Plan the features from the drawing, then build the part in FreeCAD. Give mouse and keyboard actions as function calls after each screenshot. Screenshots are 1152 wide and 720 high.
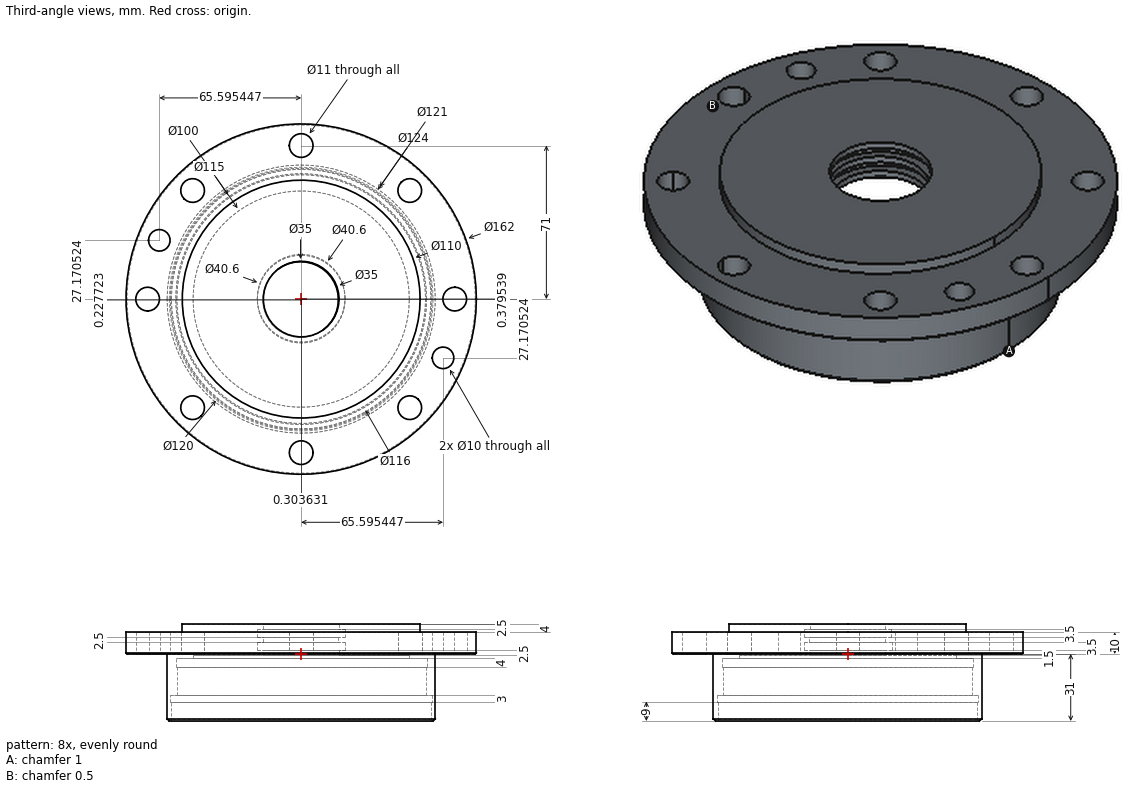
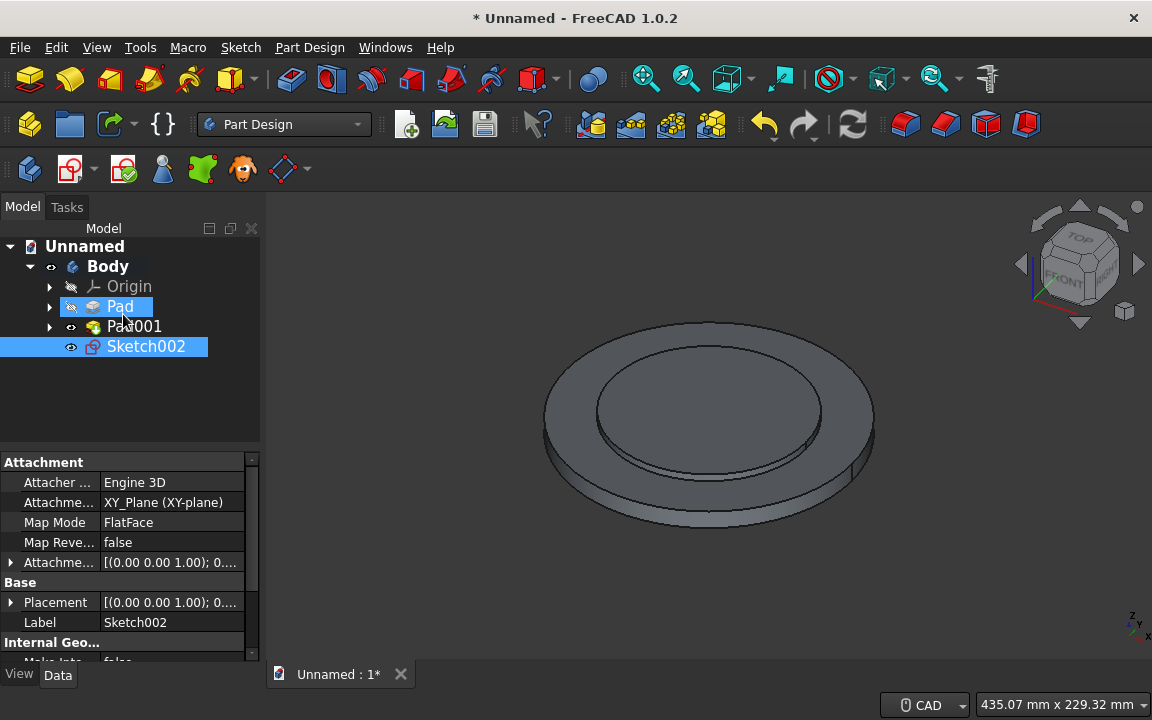
click(30, 80)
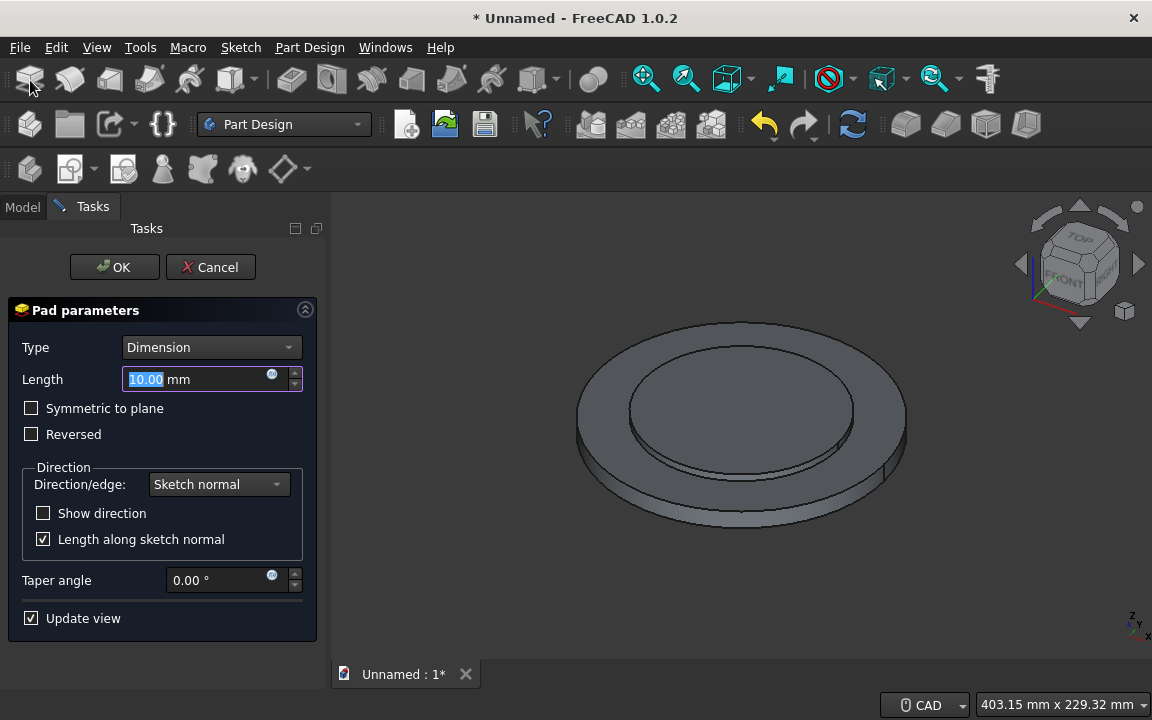
text(31)
key(Tab)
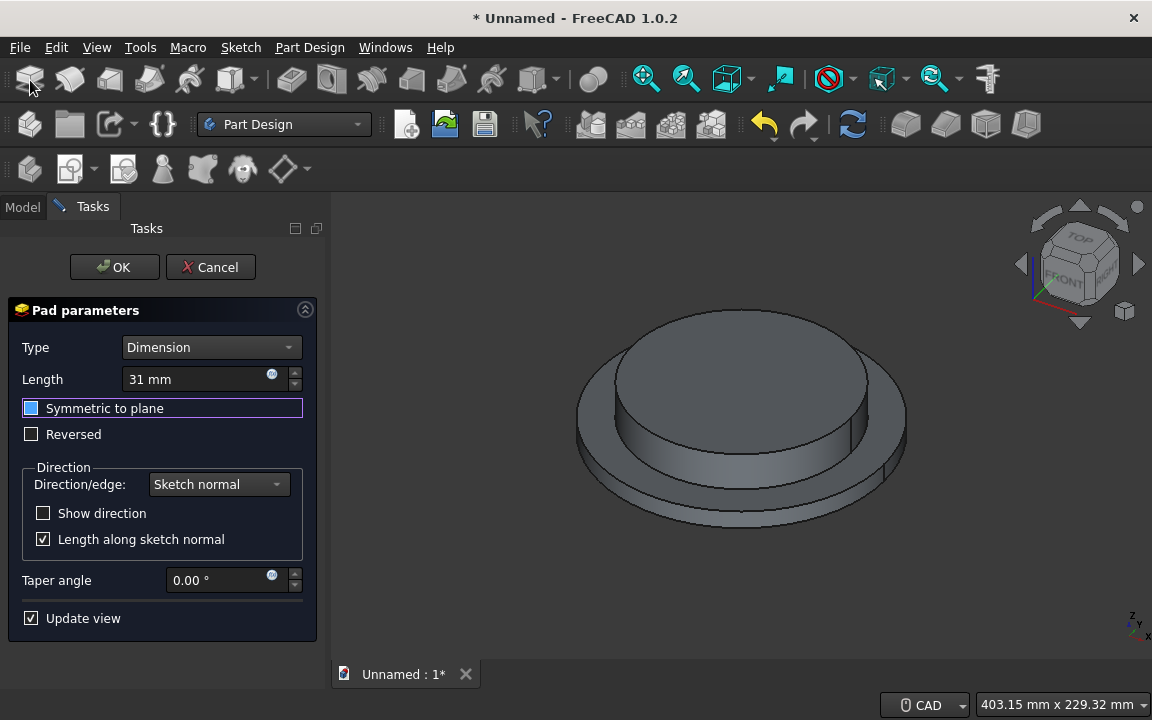
click(30, 434)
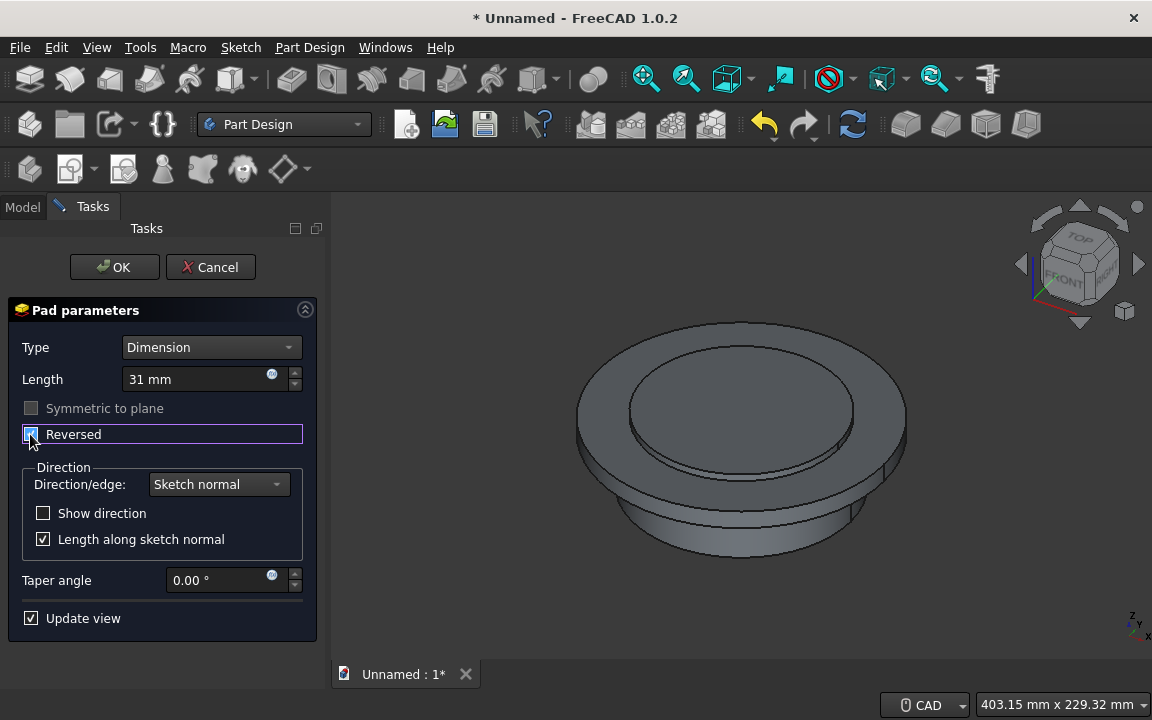
click(115, 267)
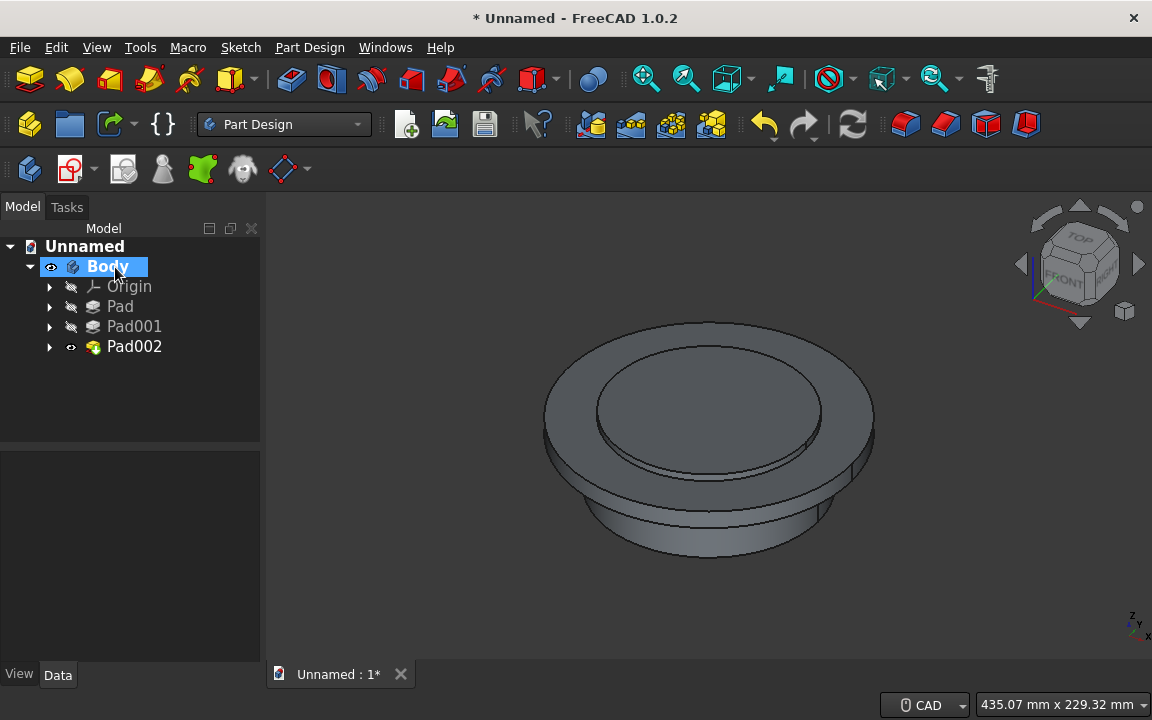
click(709, 409)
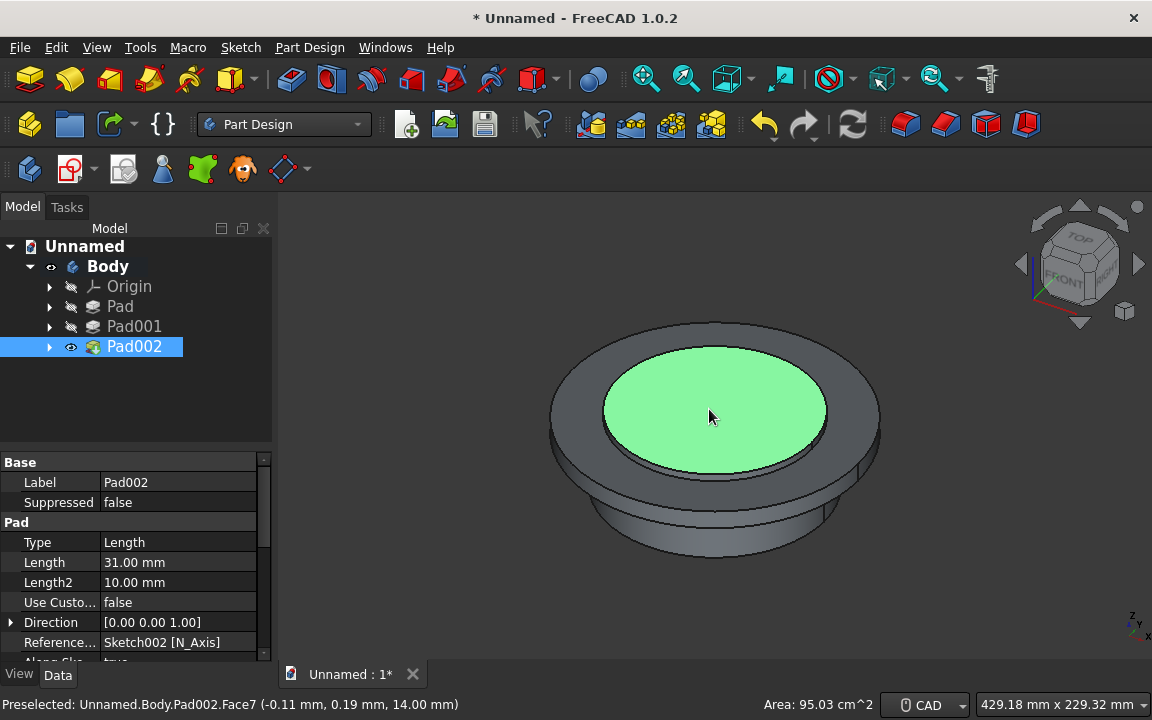
click(70, 170)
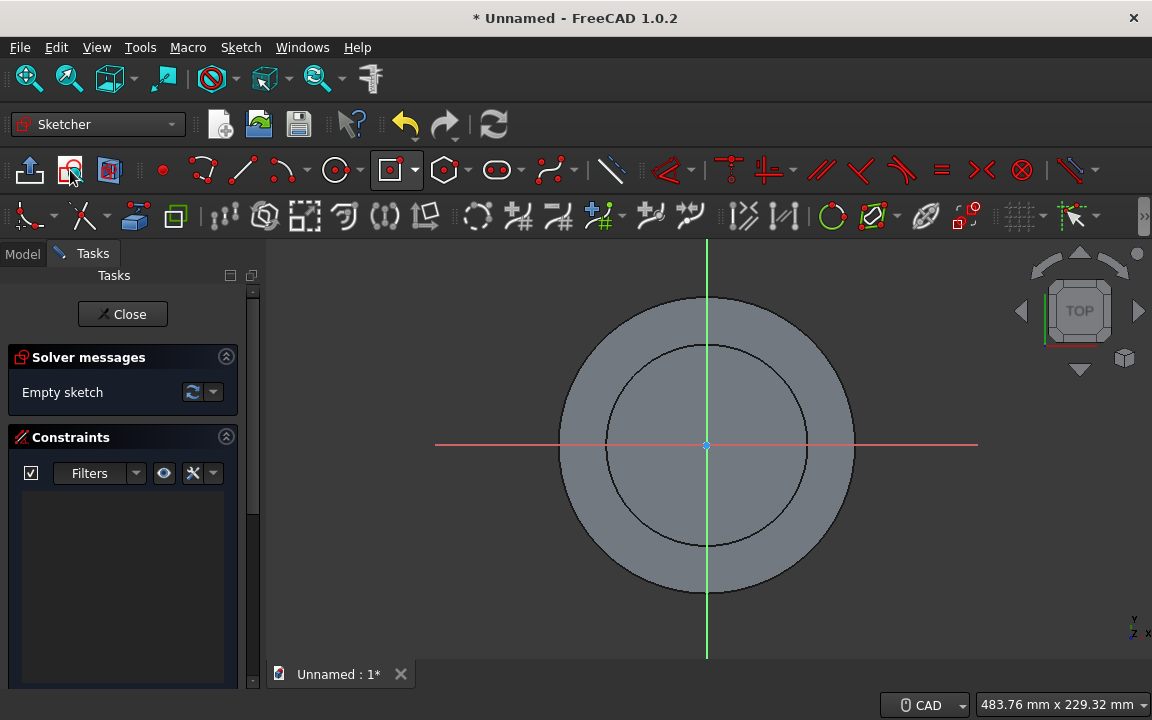
scroll(729, 444, up, 7)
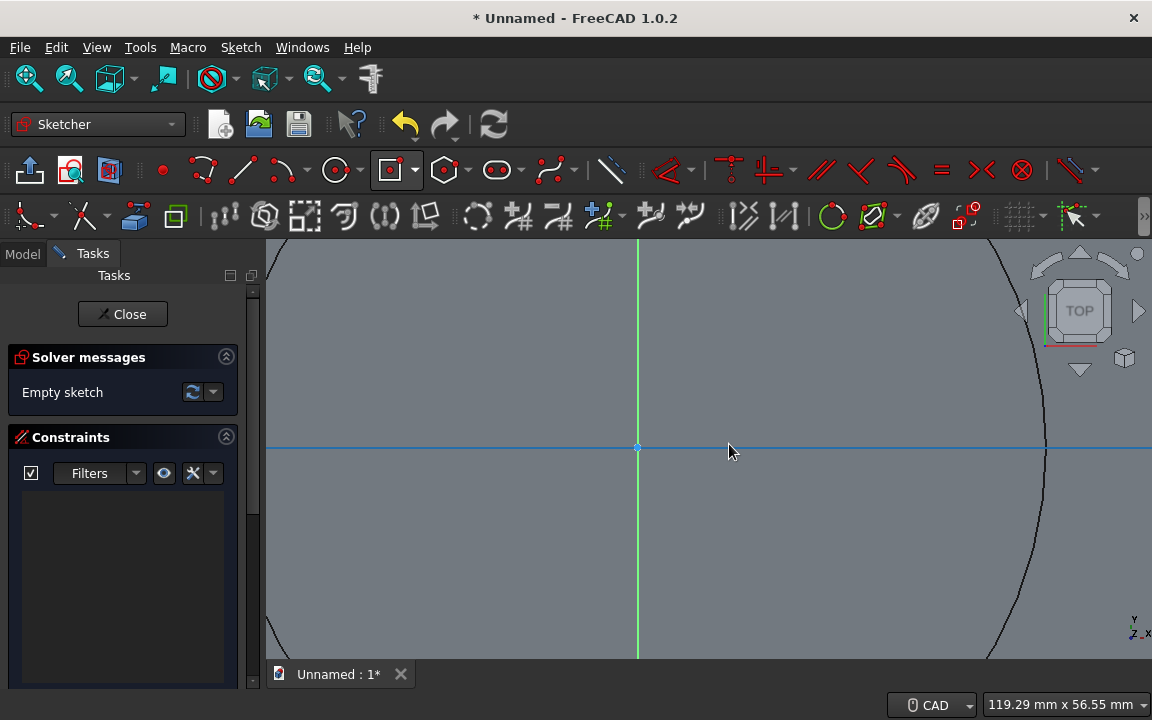
click(336, 170)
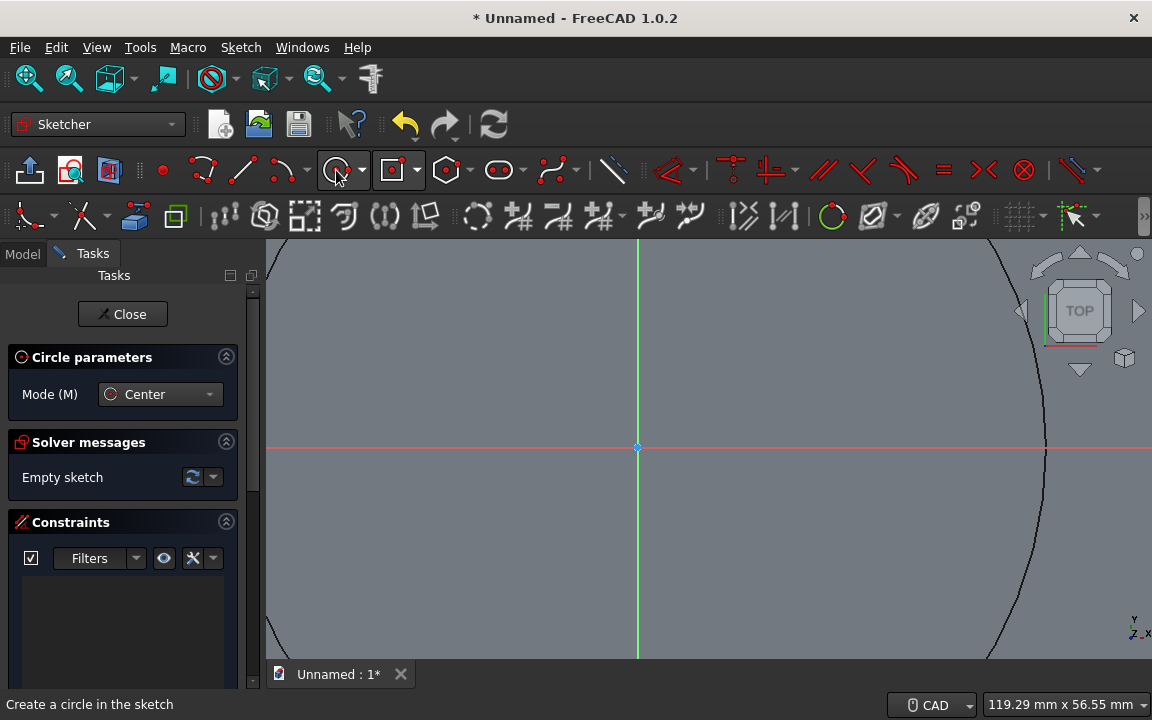
click(638, 448)
click(729, 356)
key(Escape)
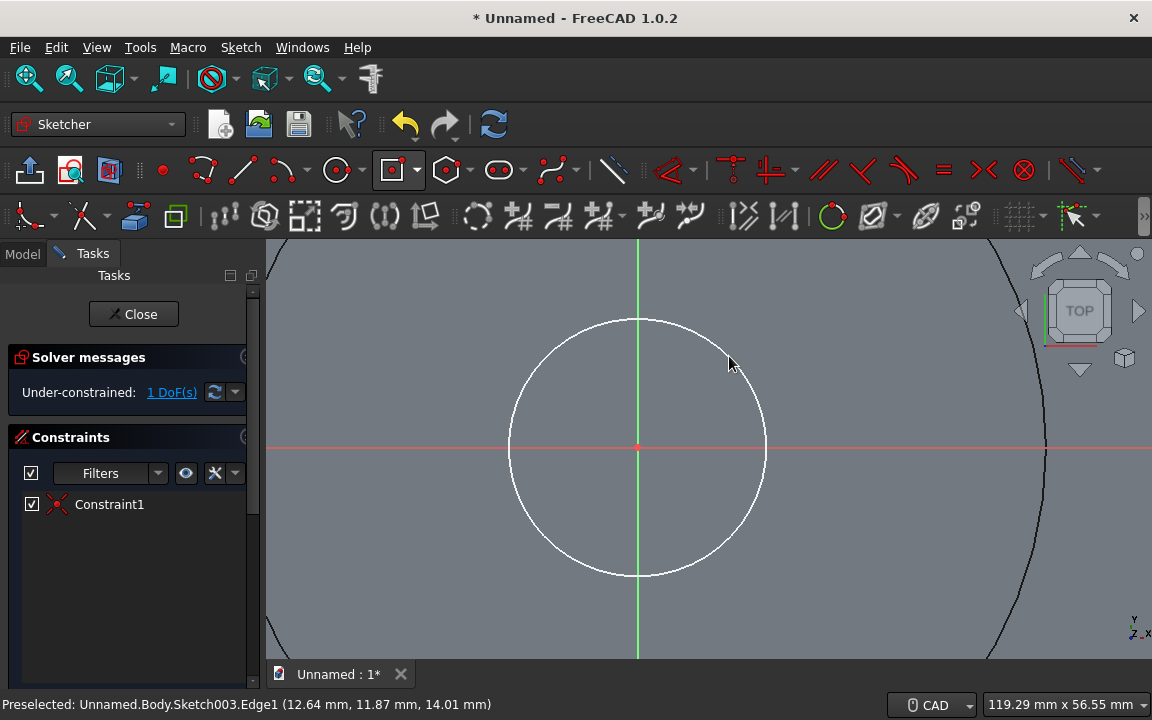
click(668, 170)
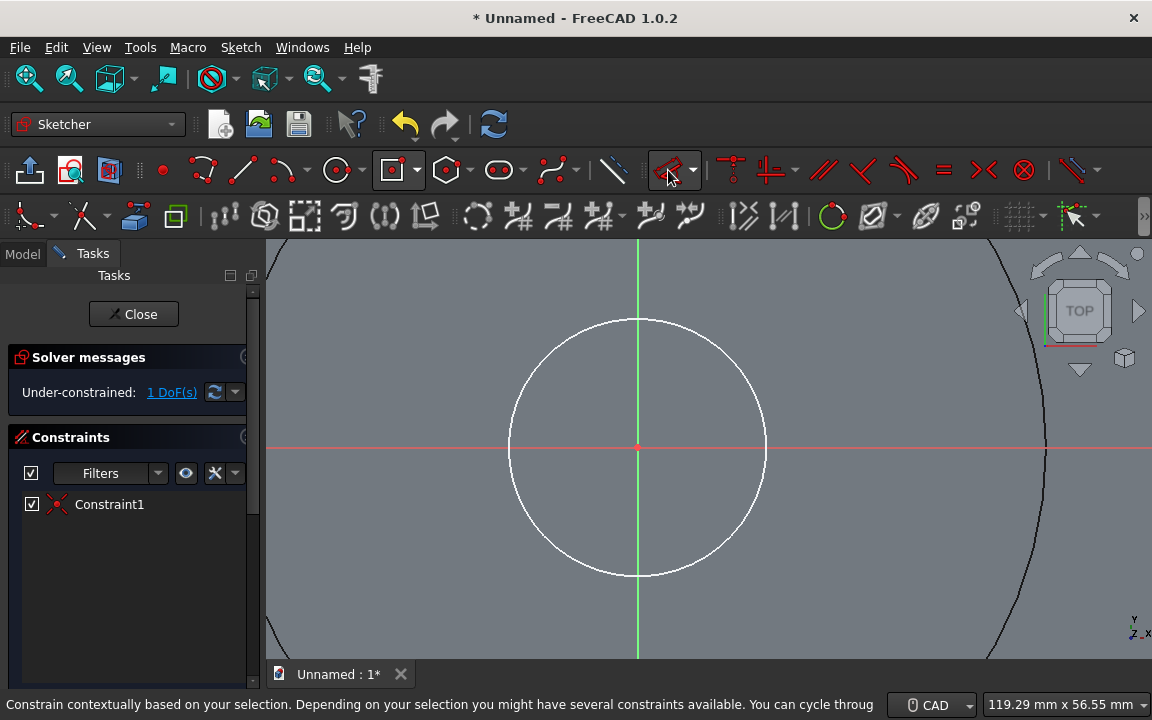
click(728, 356)
click(750, 333)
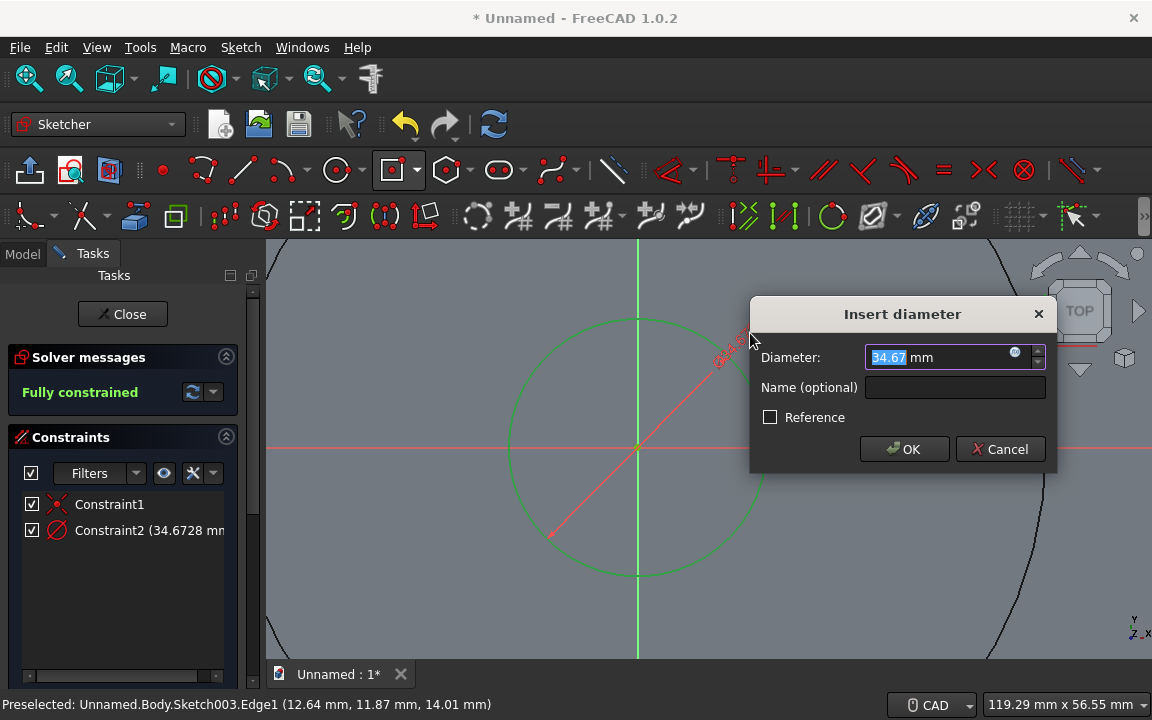
text(35)
key(Return)
key(Escape)